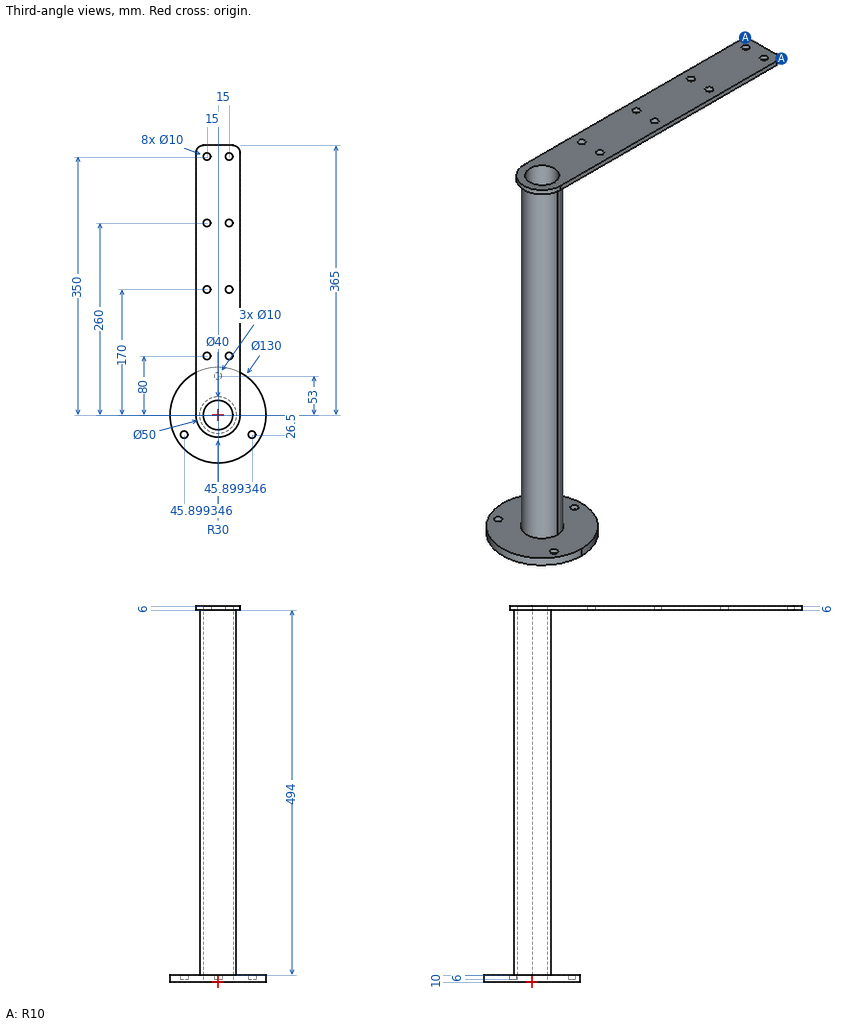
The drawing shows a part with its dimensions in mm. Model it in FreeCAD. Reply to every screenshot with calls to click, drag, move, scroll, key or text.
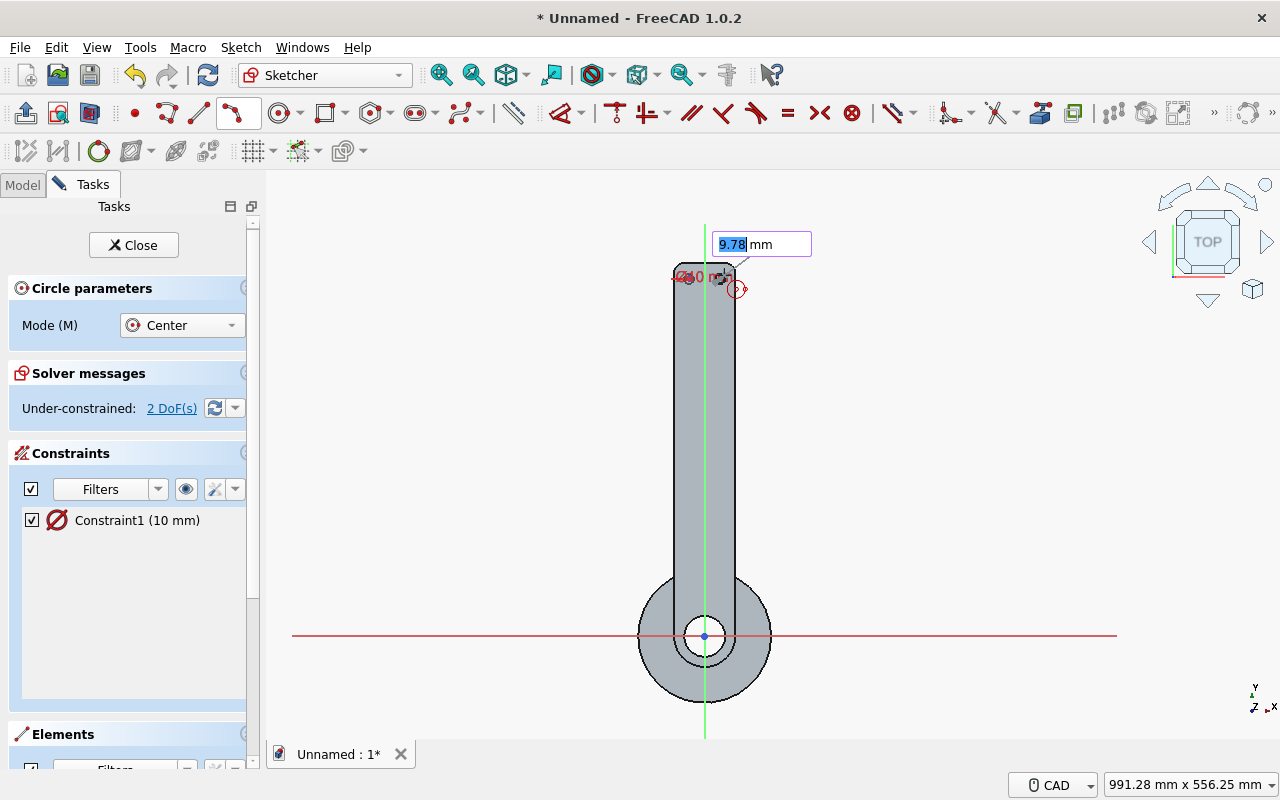
text(10)
key(Return)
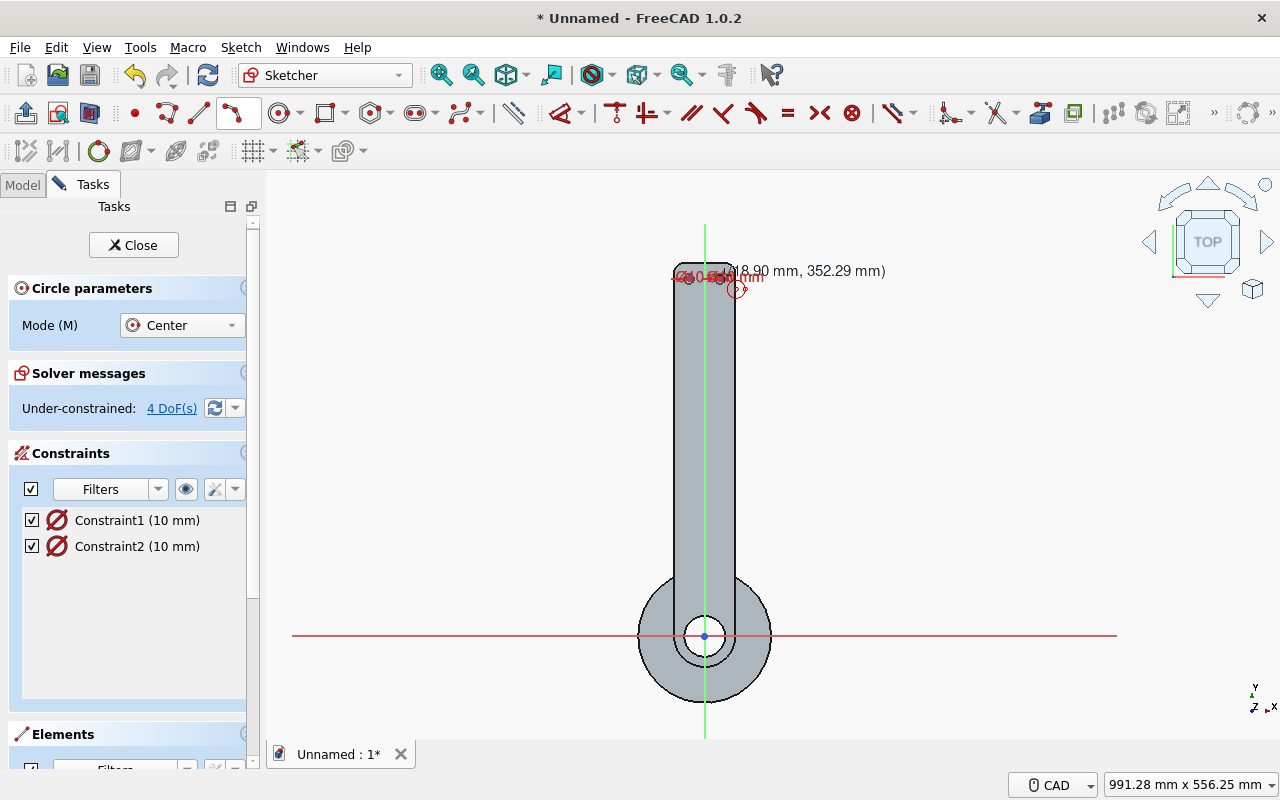
scroll(689, 370, up, 8)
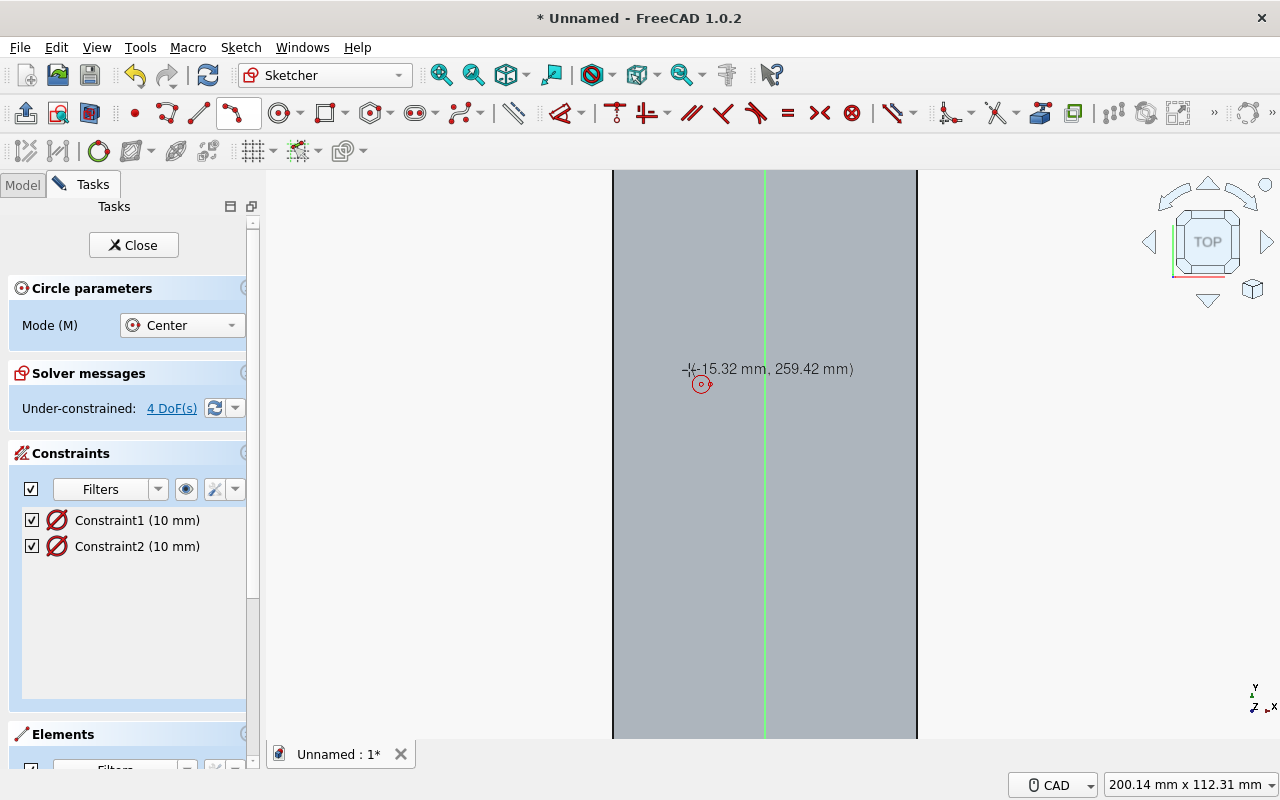
scroll(689, 370, down, 8)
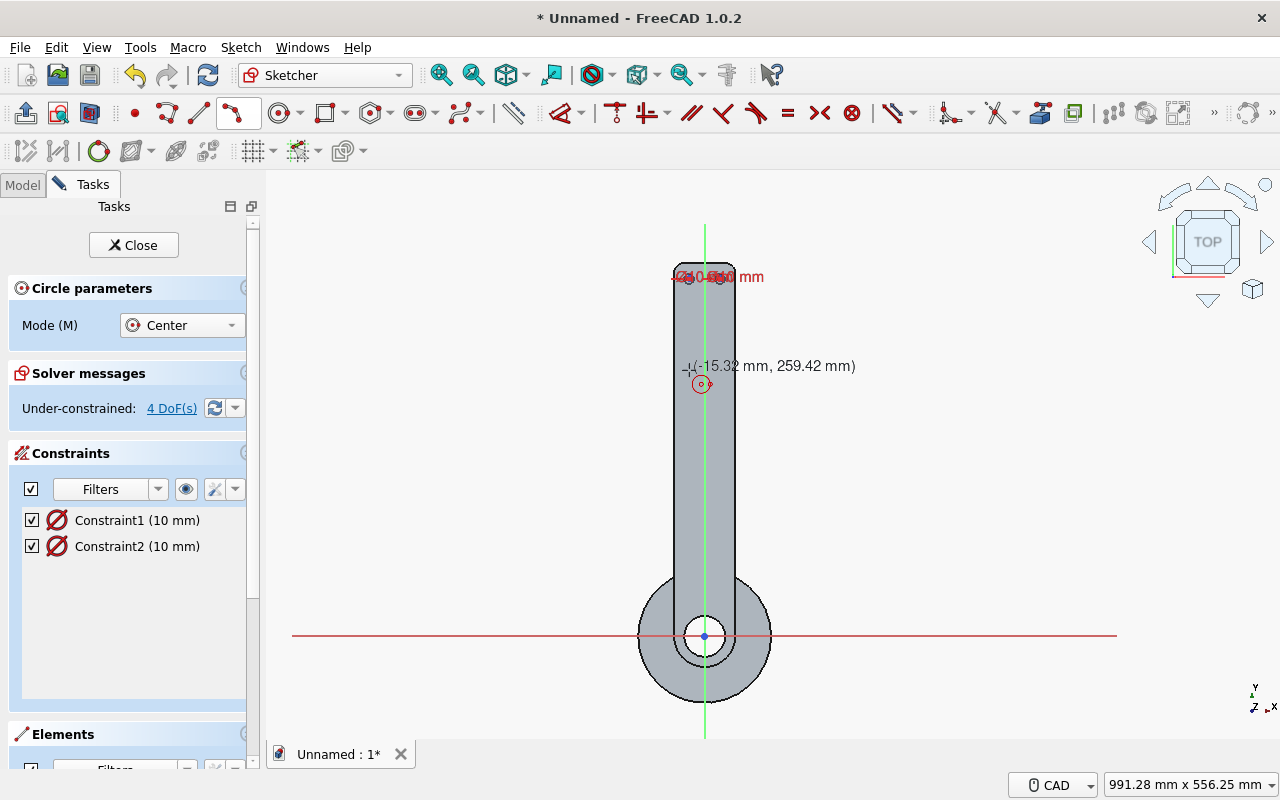
click(689, 370)
move(686, 367)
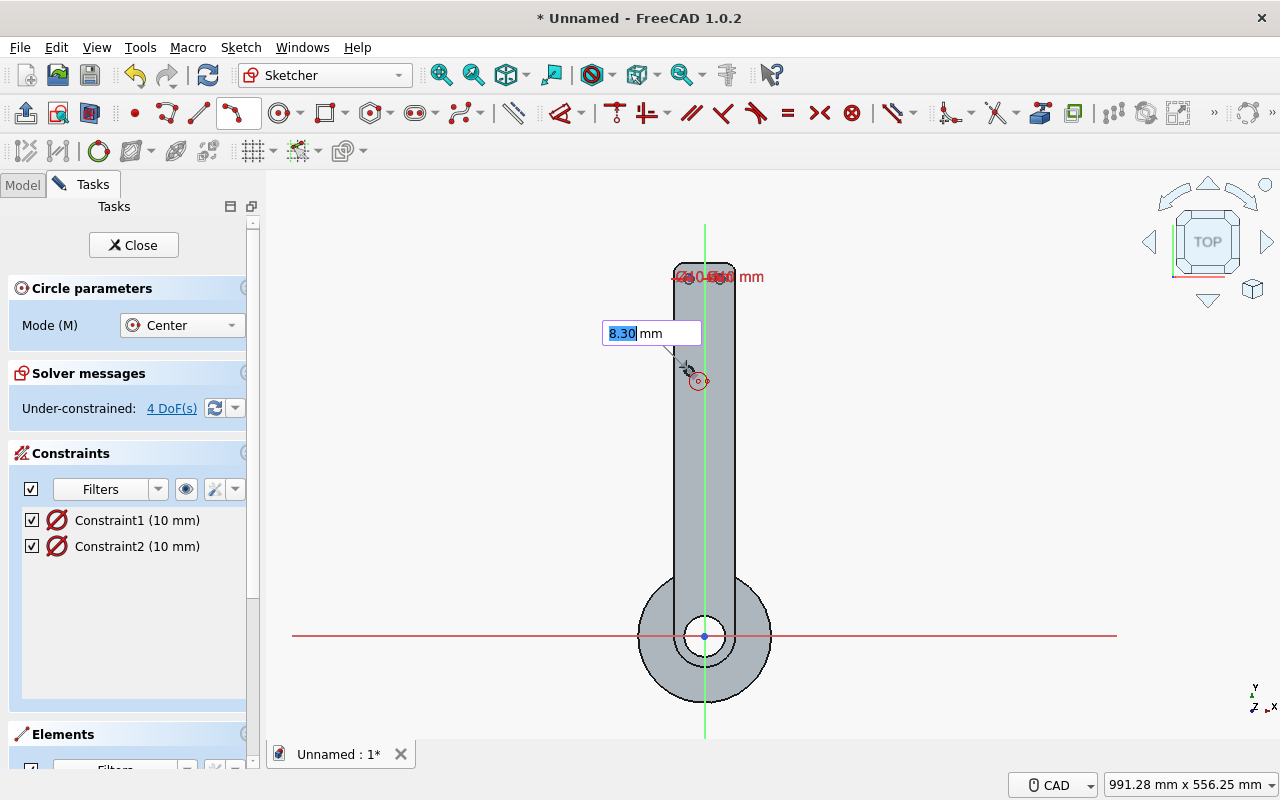
text(10)
key(Return)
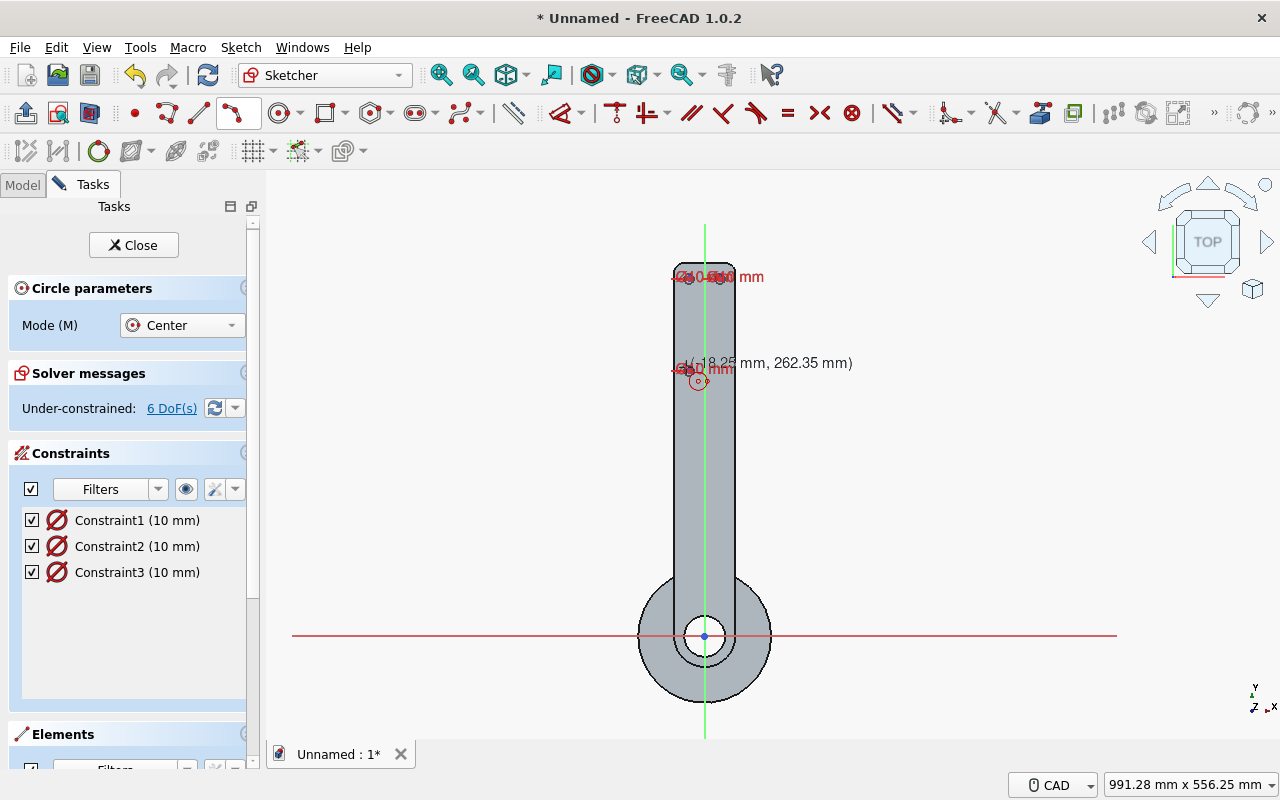
scroll(720, 370, up, 8)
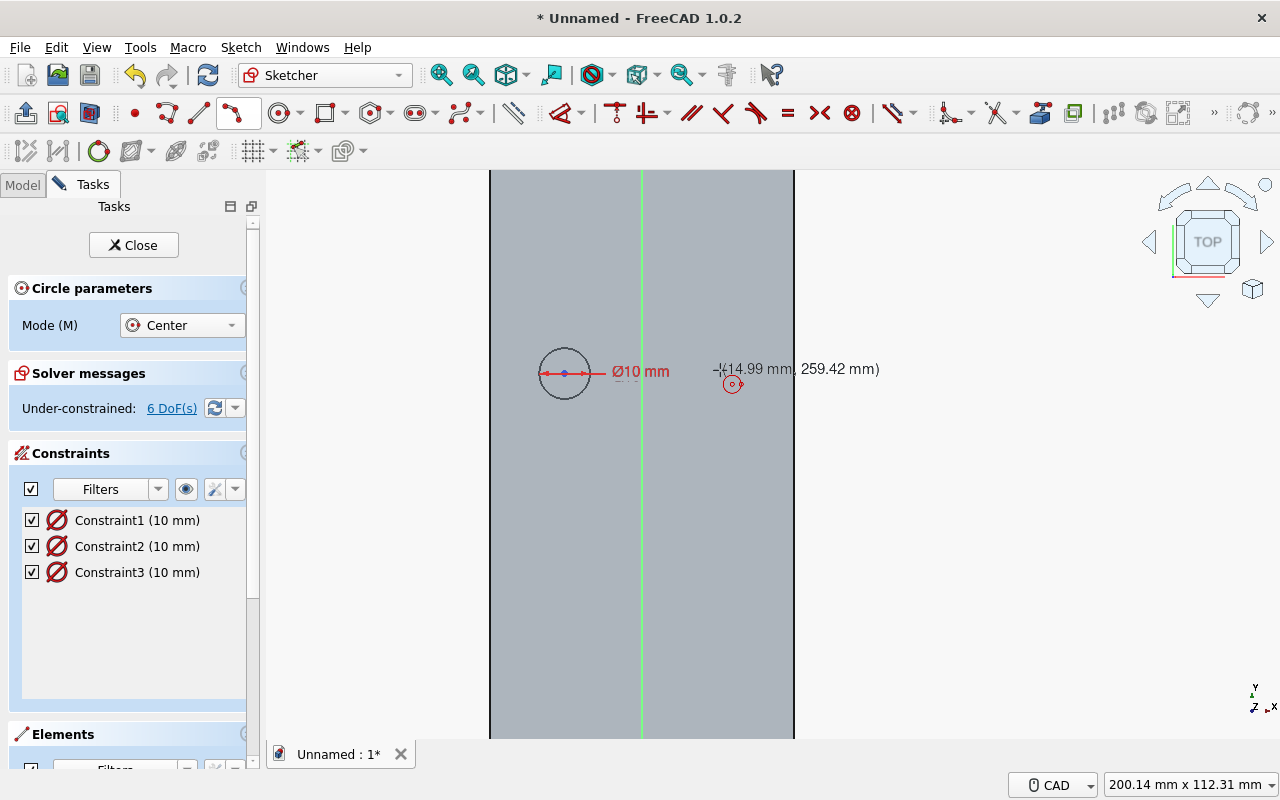
scroll(720, 370, down, 8)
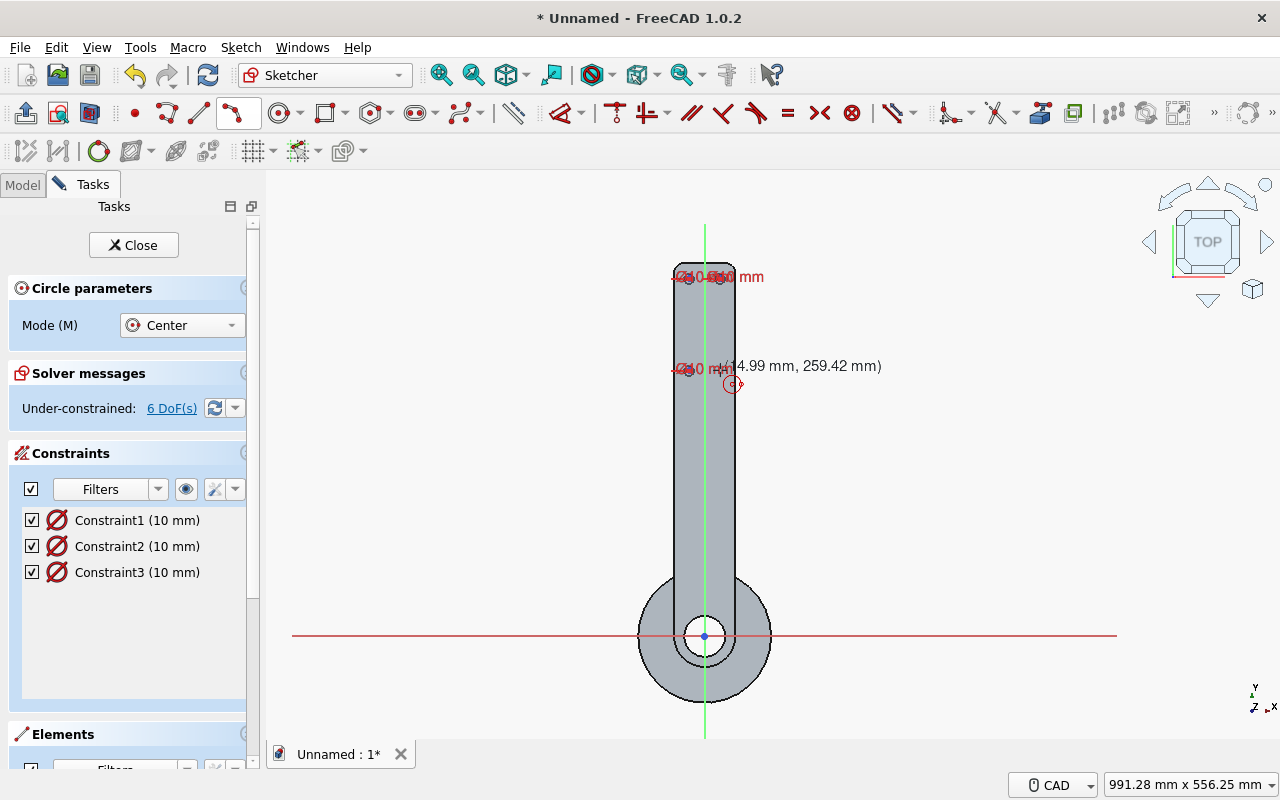
click(720, 370)
move(724, 367)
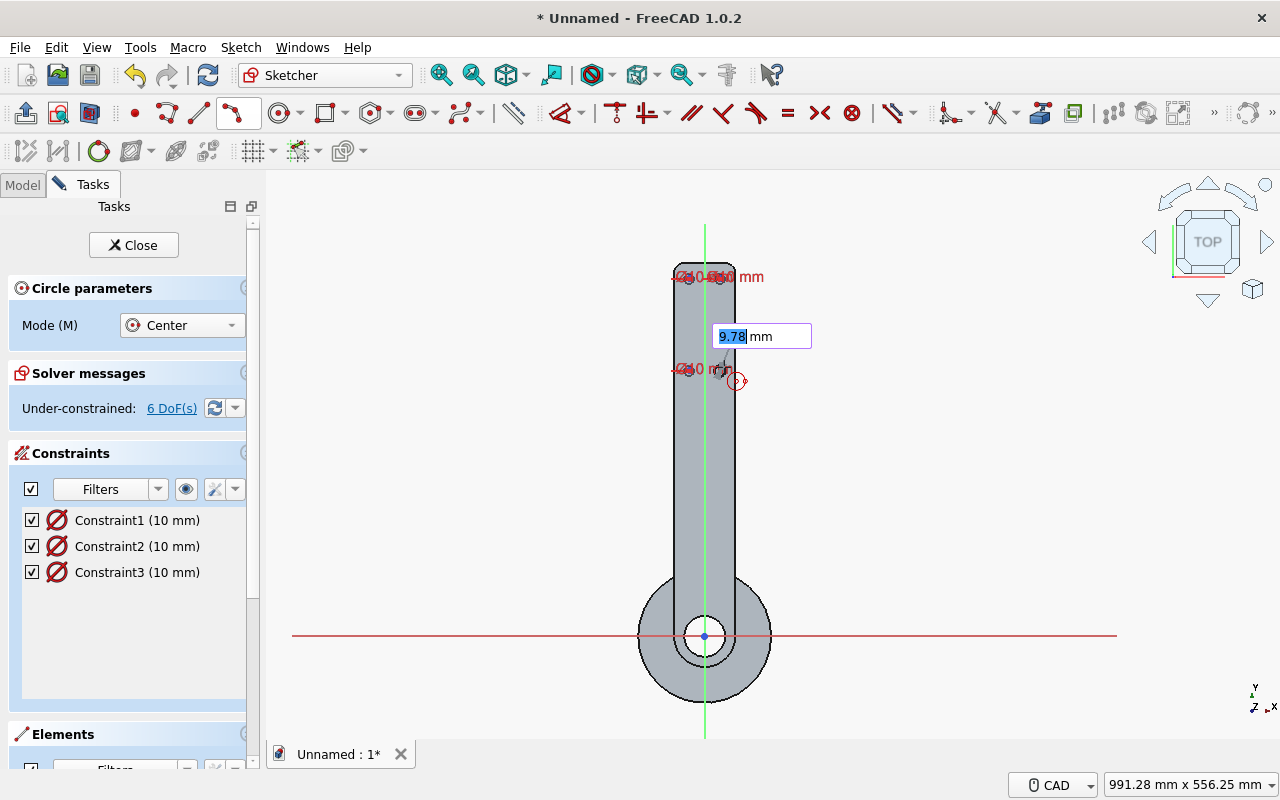
text(10)
key(Return)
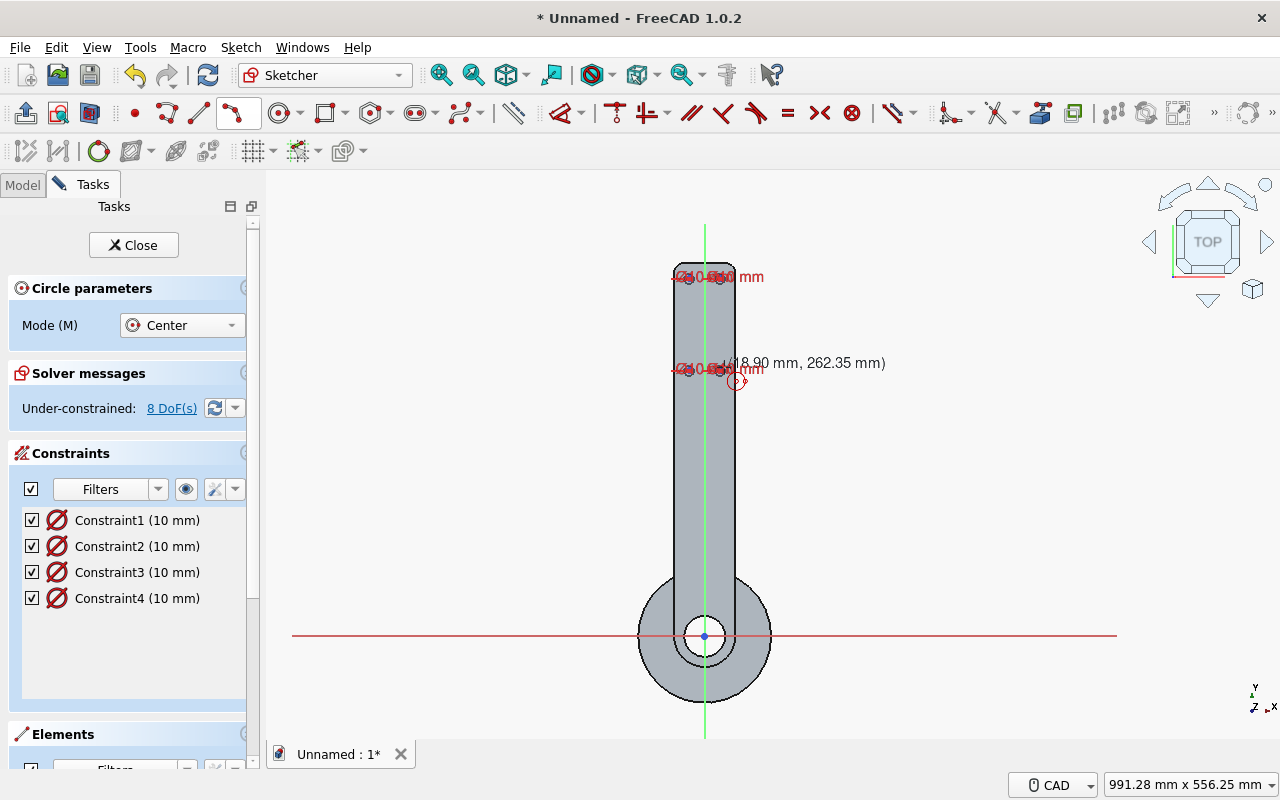
scroll(689, 462, up, 8)